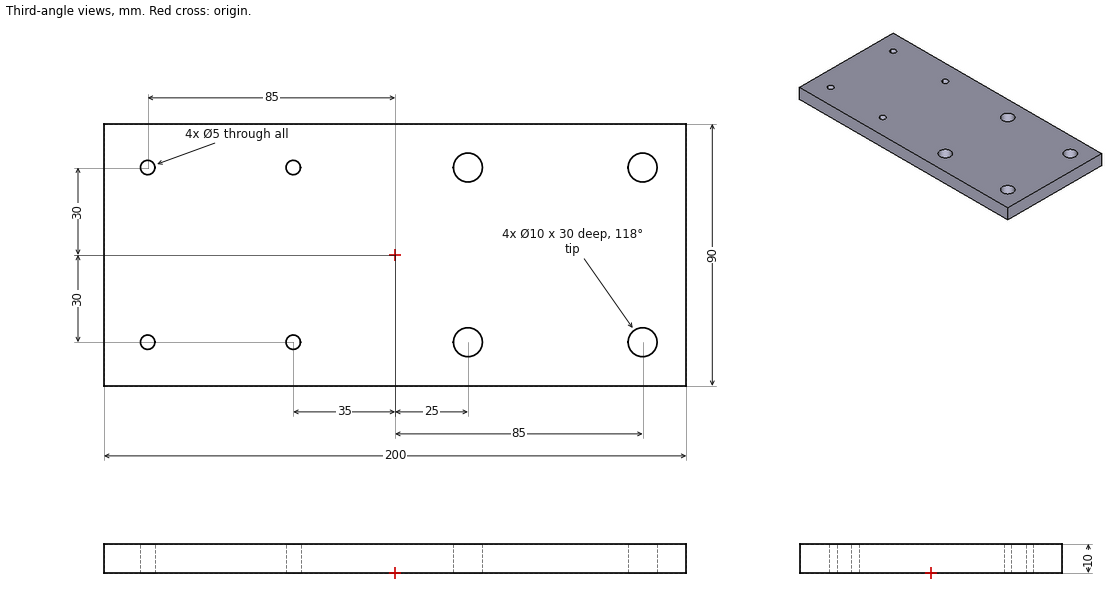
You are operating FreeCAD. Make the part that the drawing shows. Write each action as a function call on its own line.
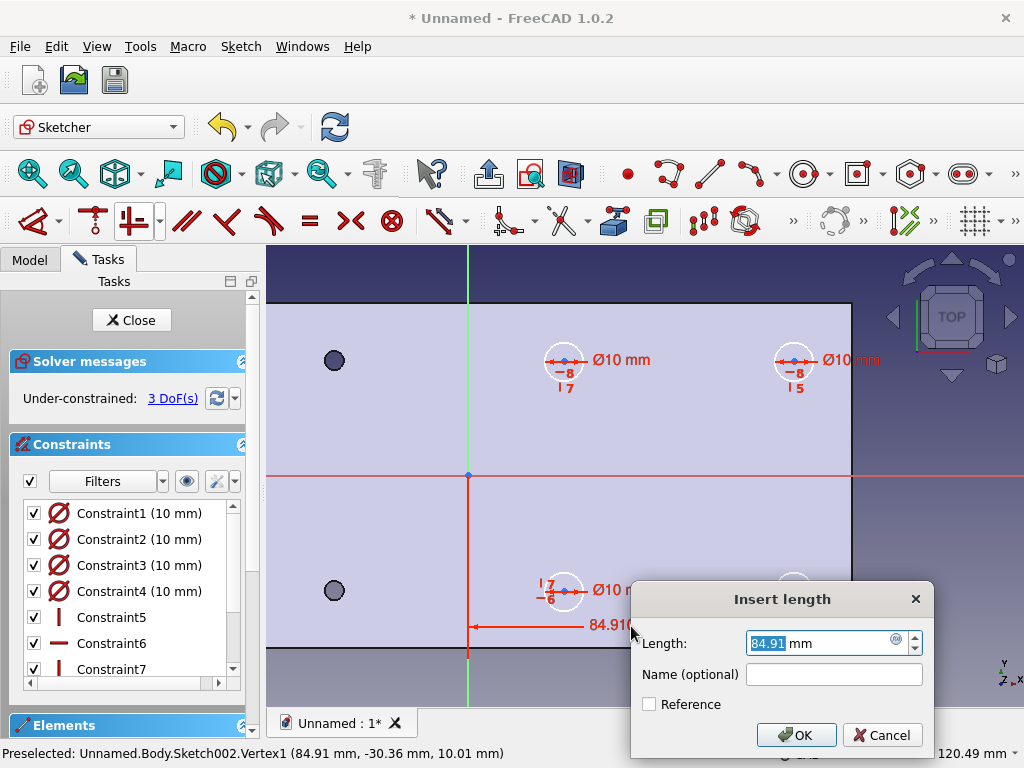
text(85)
key(Return)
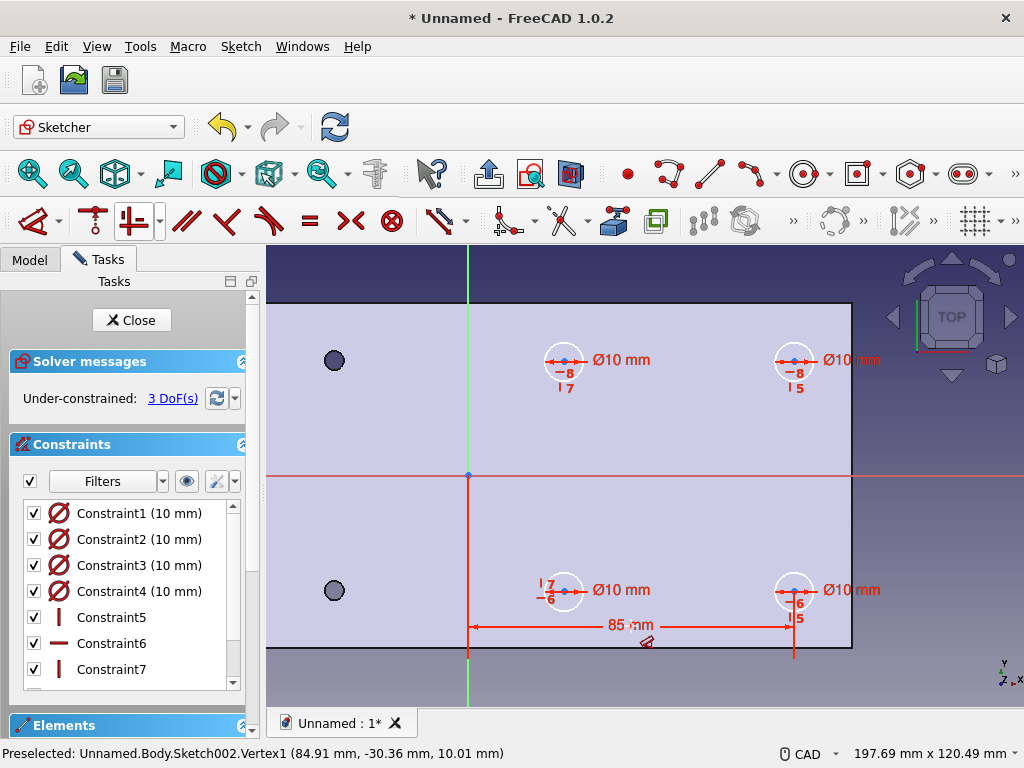
click(794, 592)
click(434, 534)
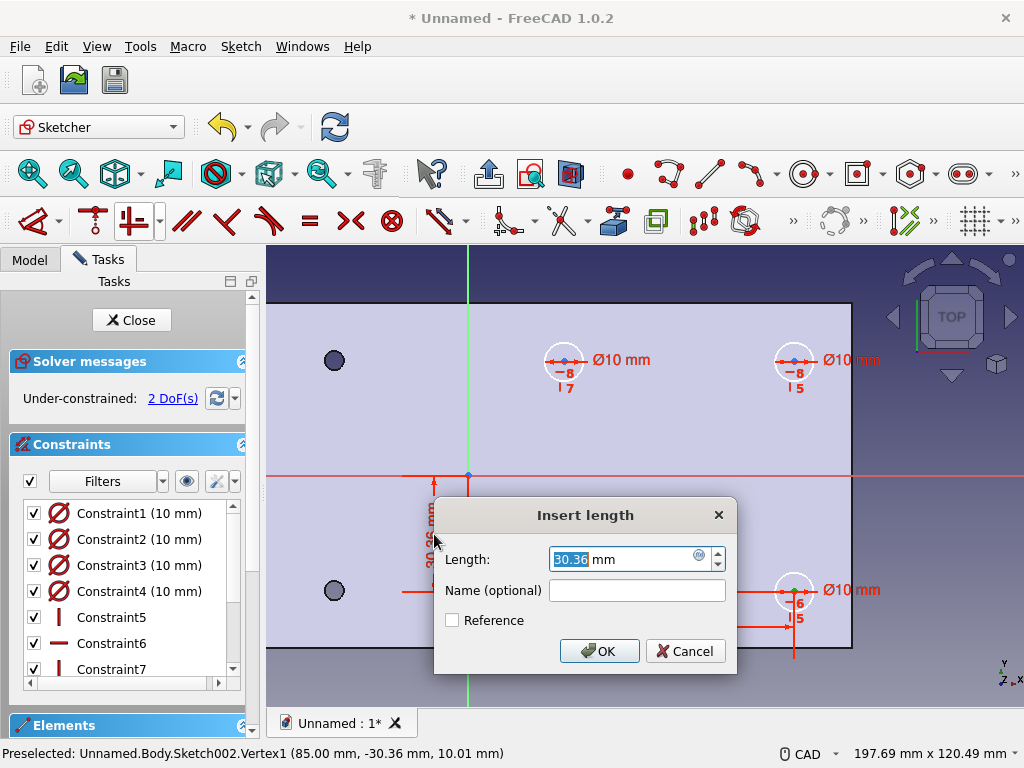
text(30)
key(Return)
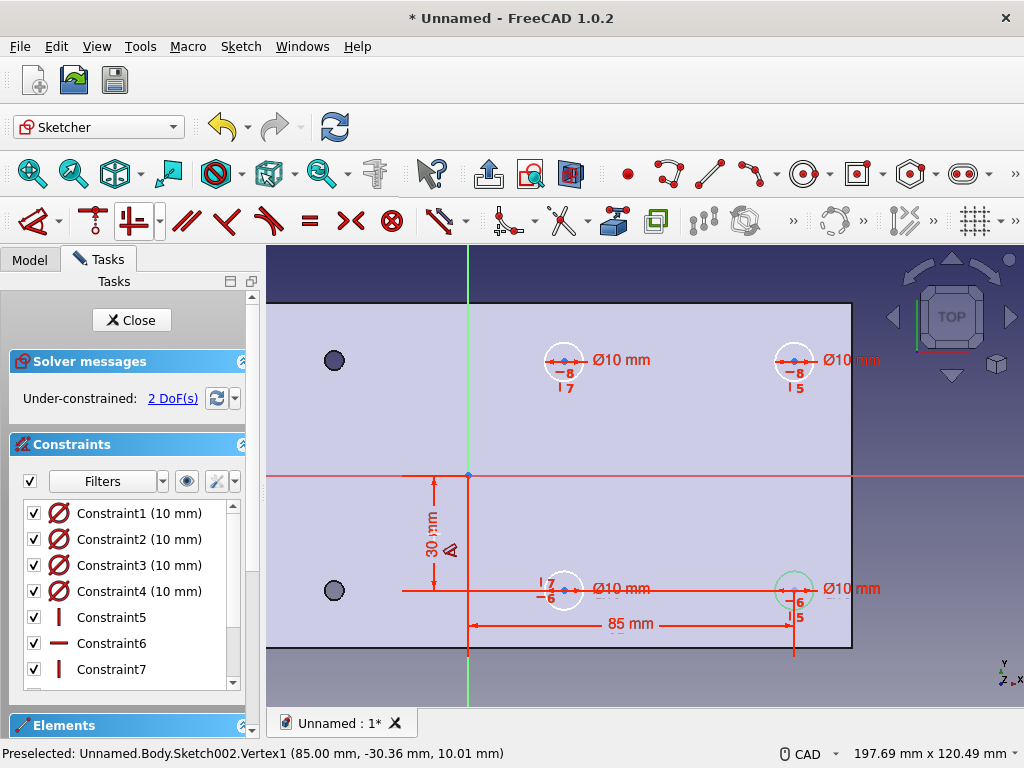
click(794, 362)
click(434, 419)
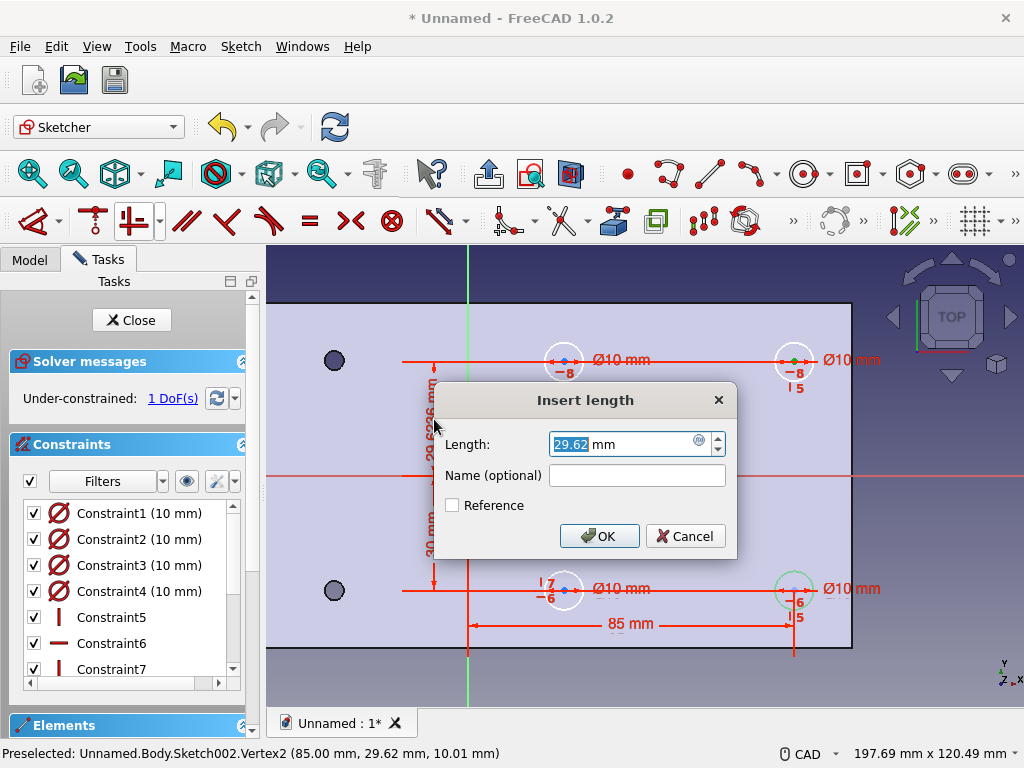
text(30)
key(Return)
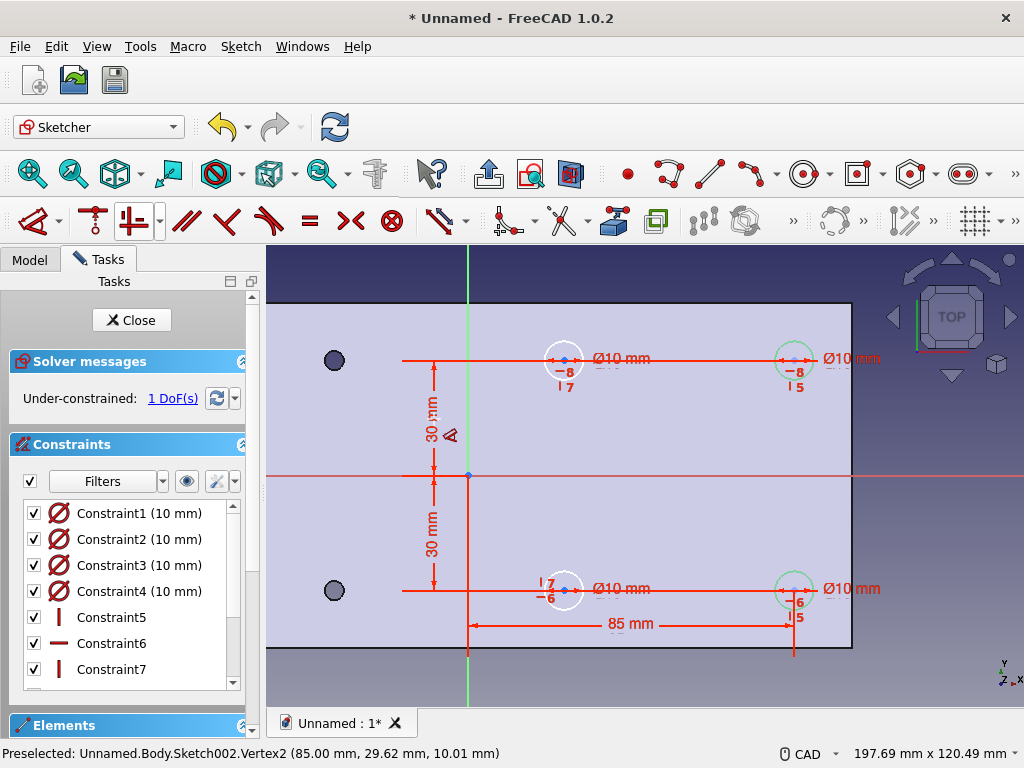
click(564, 591)
click(516, 625)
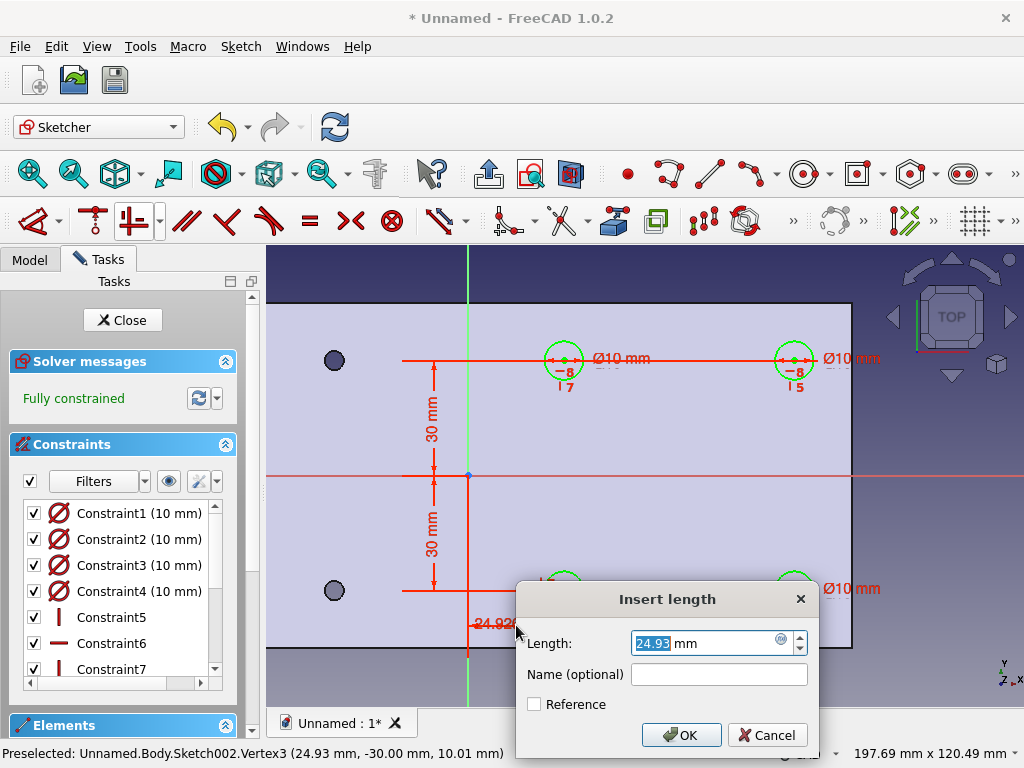
text(25)
key(Return)
key(Escape)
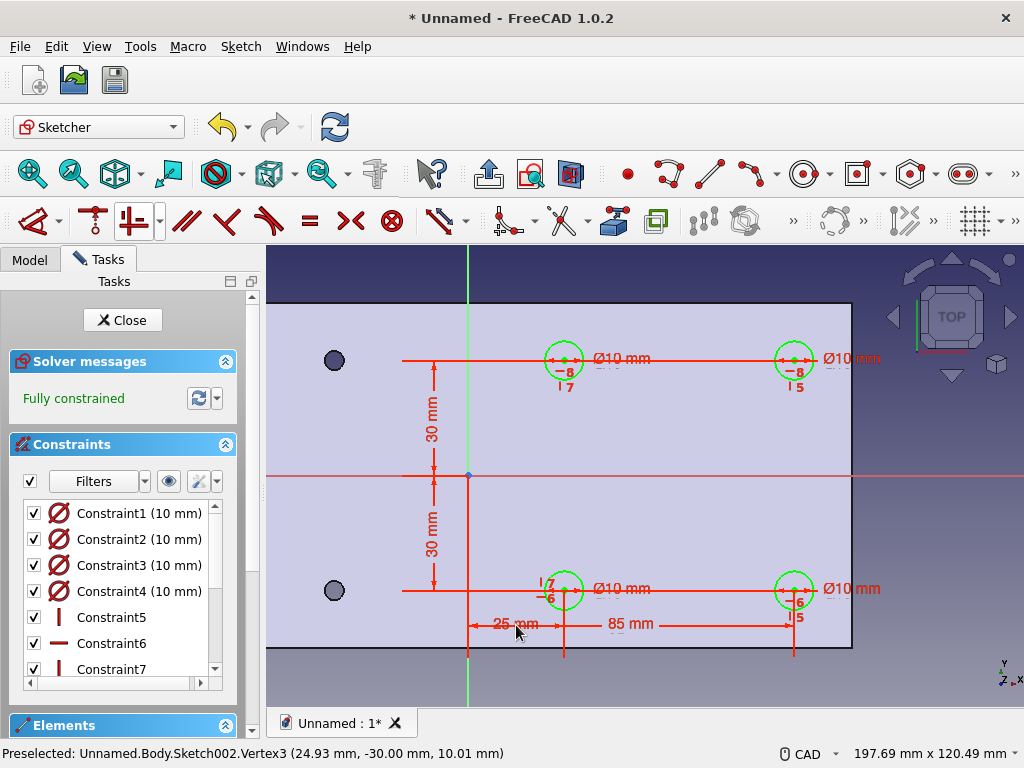
click(123, 320)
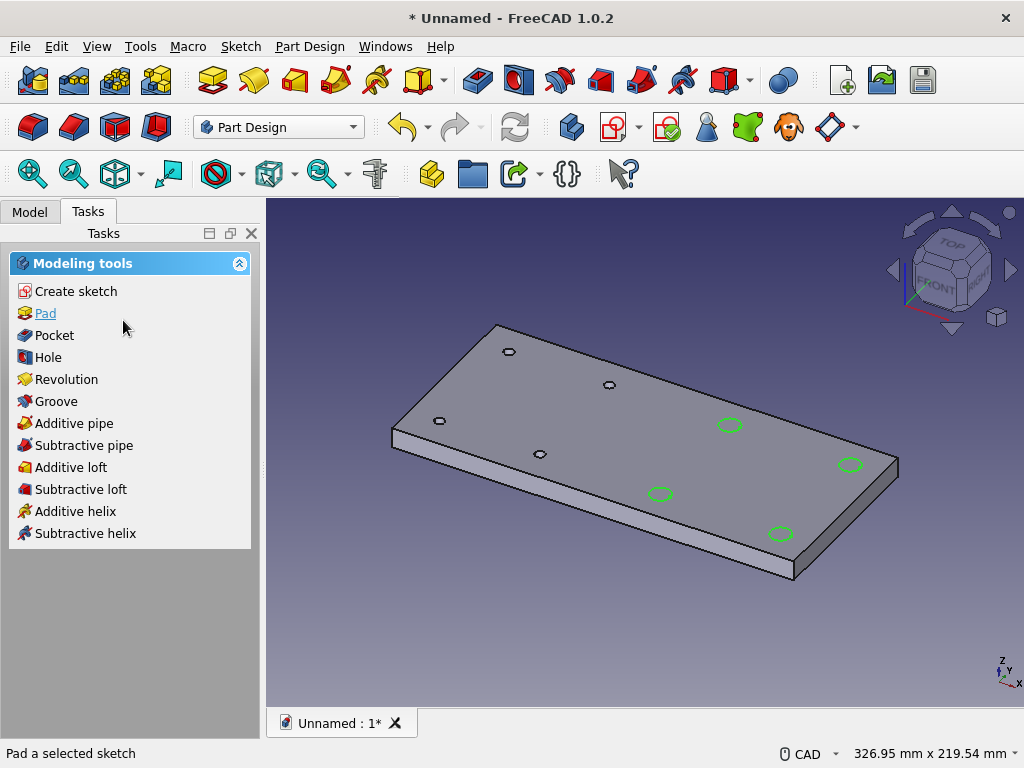
click(519, 80)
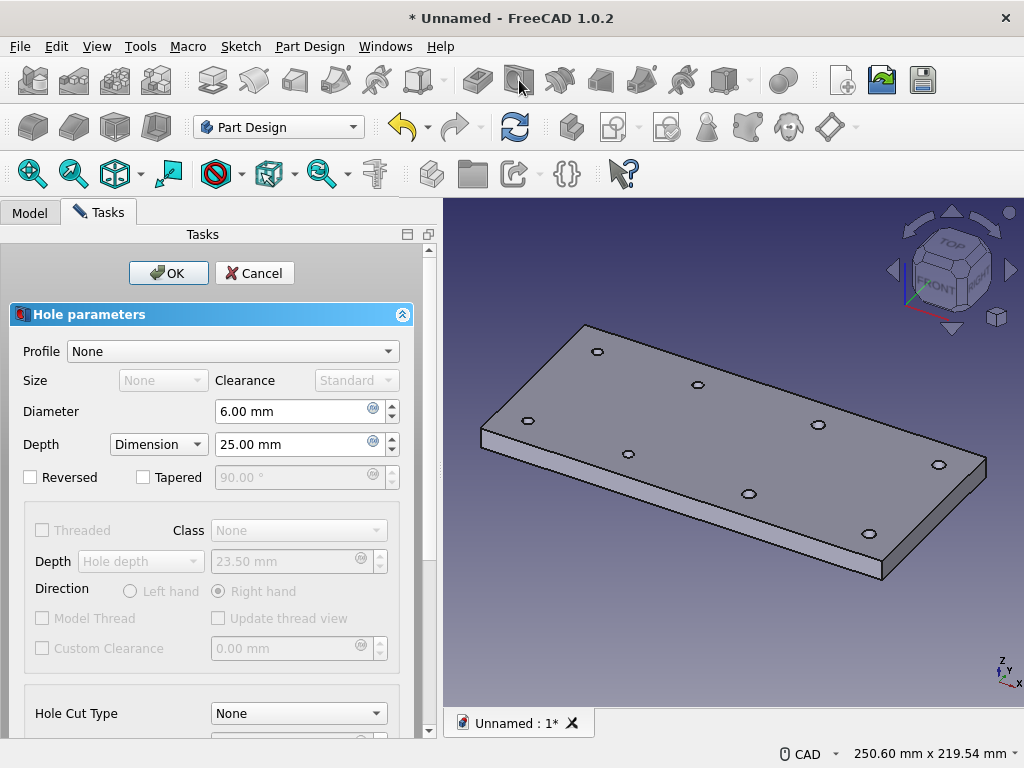
triple_click(300, 412)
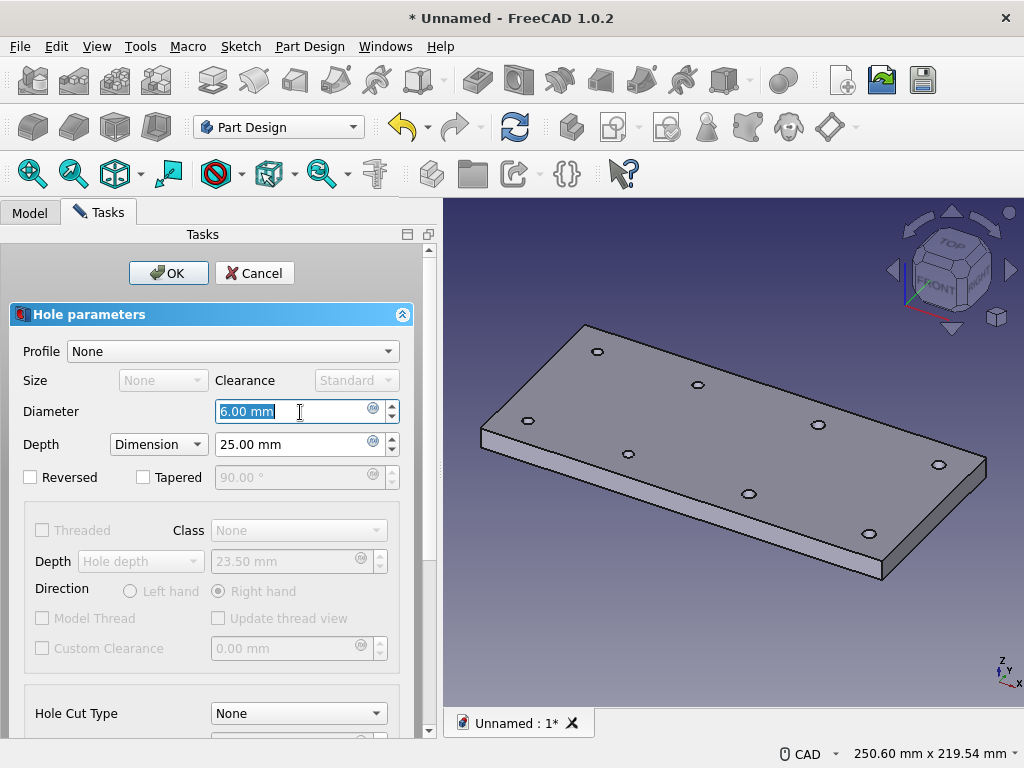
text(10)
key(Tab)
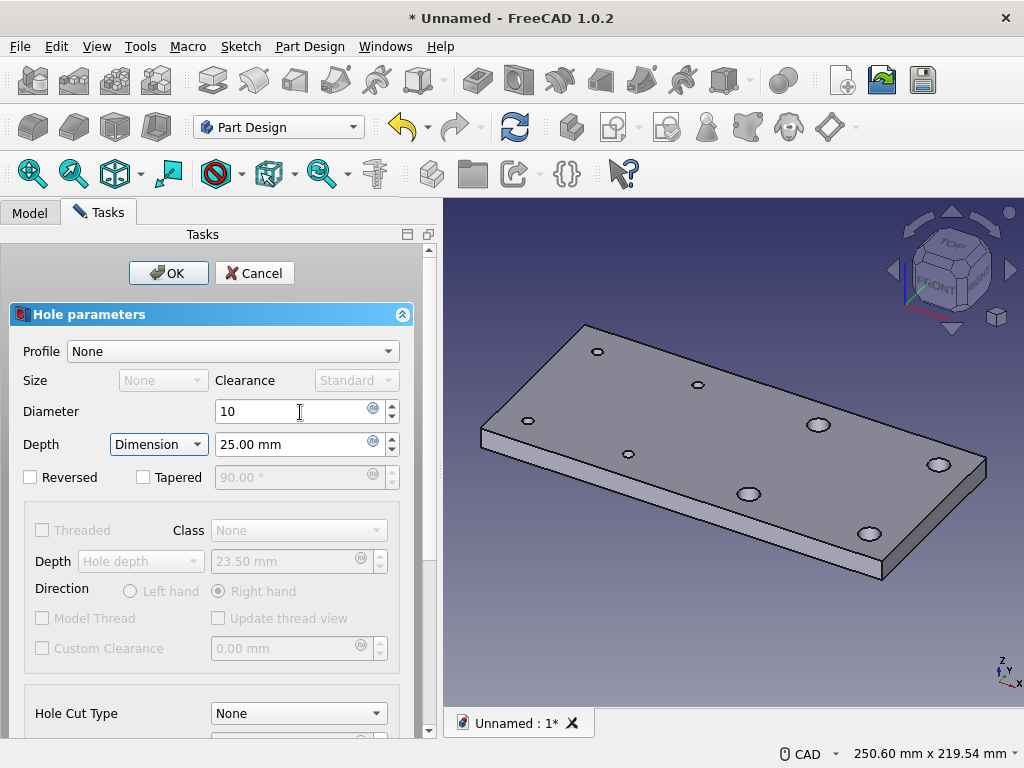
triple_click(300, 444)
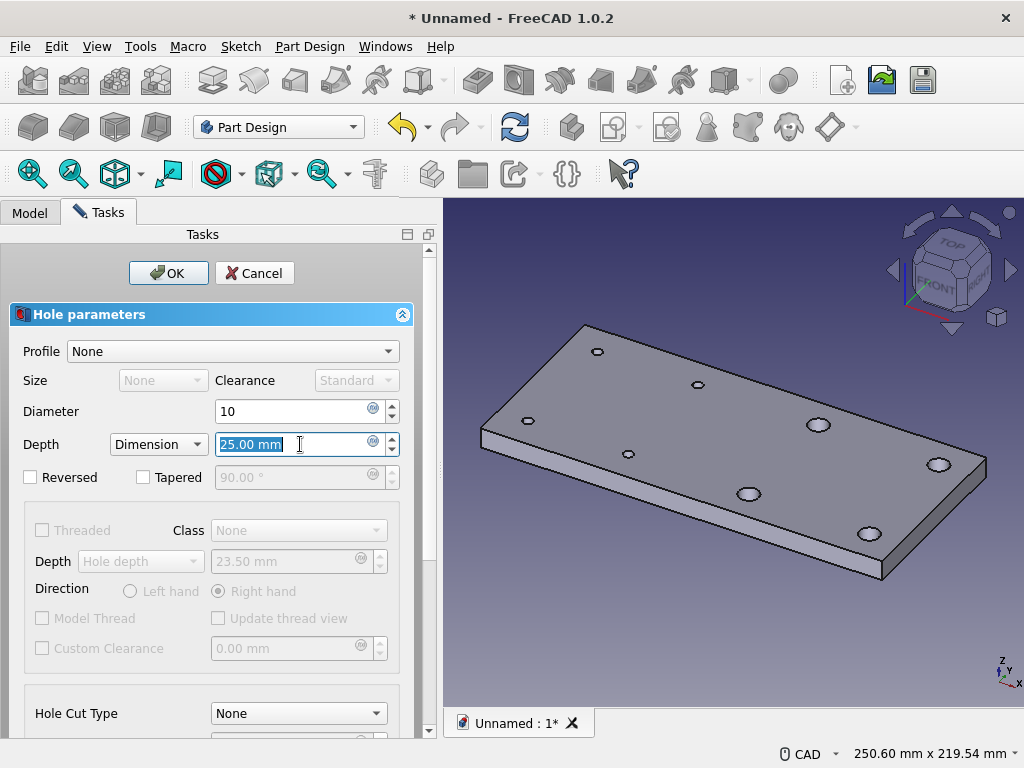
text(30)
key(Tab)